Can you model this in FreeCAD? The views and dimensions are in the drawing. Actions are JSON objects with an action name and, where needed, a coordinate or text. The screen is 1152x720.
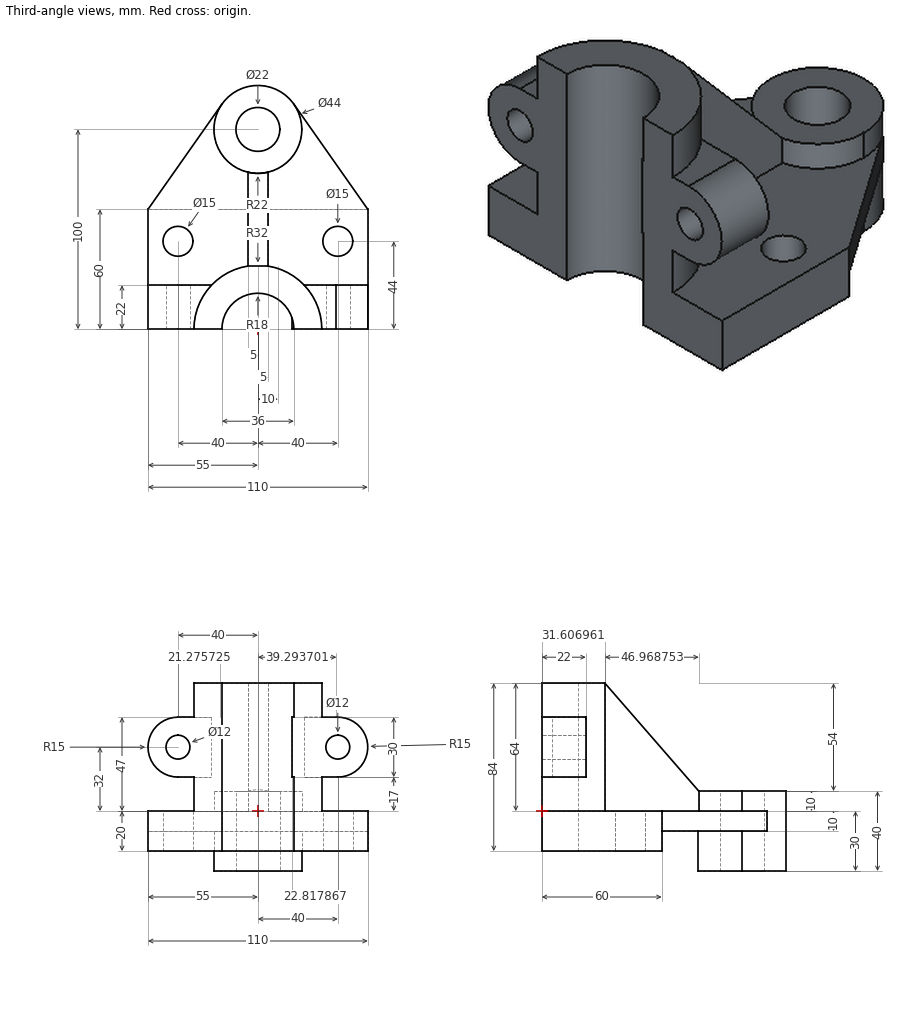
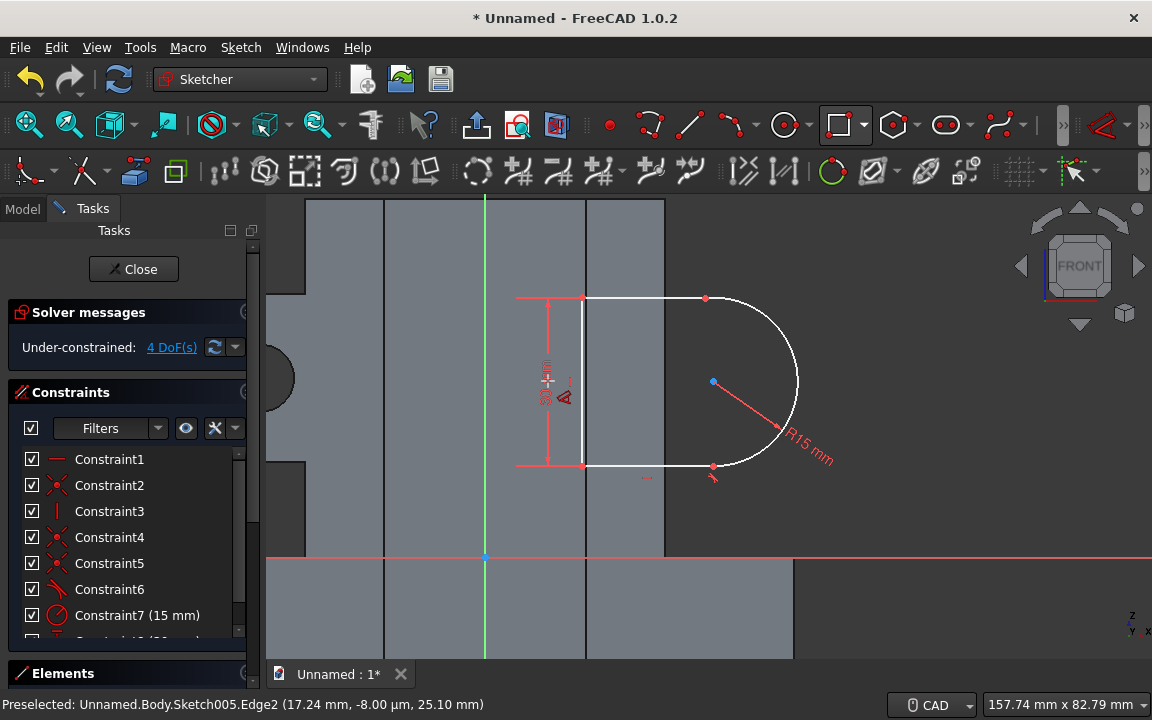
{"action": "left_click", "coordinate": [713, 466]}
{"action": "left_click", "coordinate": [599, 592]}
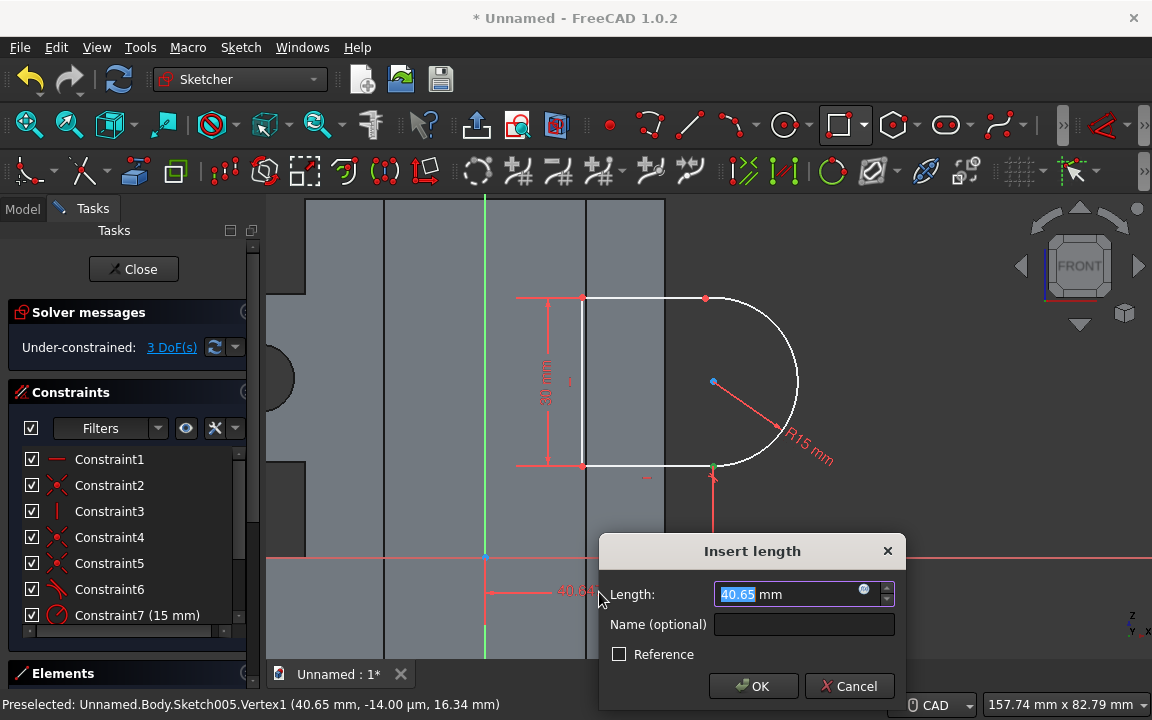
{"action": "type", "text": "40"}
{"action": "key", "text": "Return"}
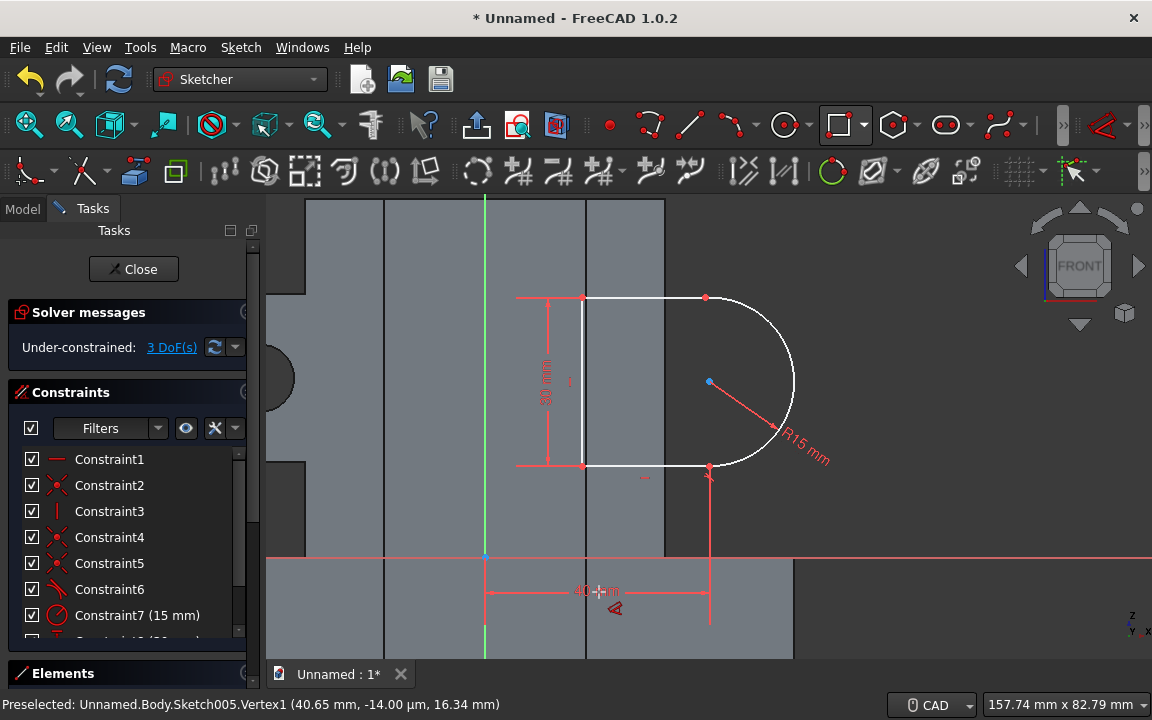
{"action": "left_click", "coordinate": [710, 466]}
{"action": "left_click", "coordinate": [451, 512]}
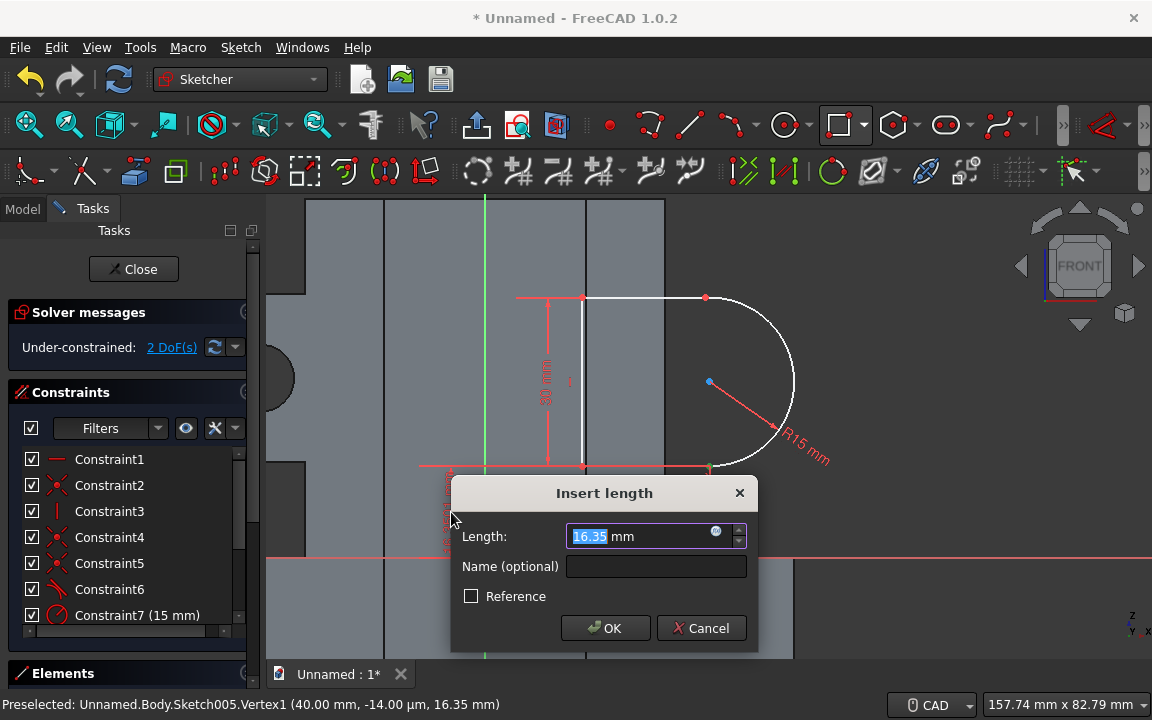
{"action": "type", "text": "17"}
{"action": "key", "text": "Return"}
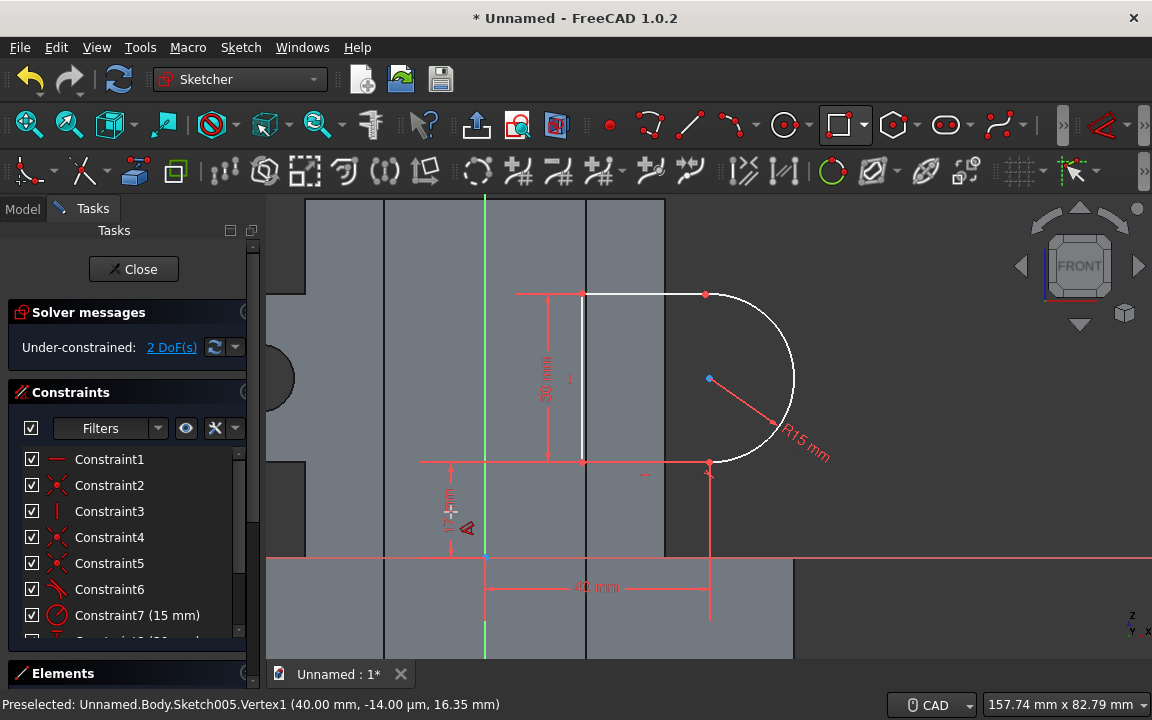
{"action": "left_click", "coordinate": [671, 462]}
{"action": "left_click", "coordinate": [646, 496]}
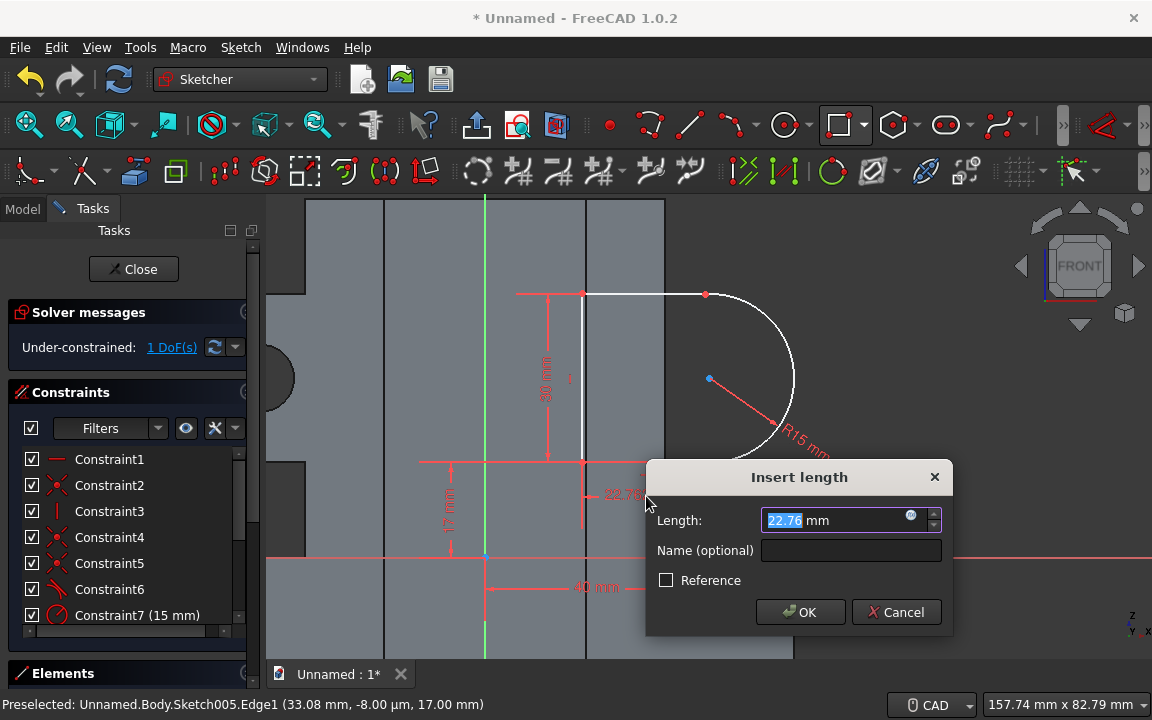
{"action": "type", "text": "22.817867"}
{"action": "key", "text": "Return"}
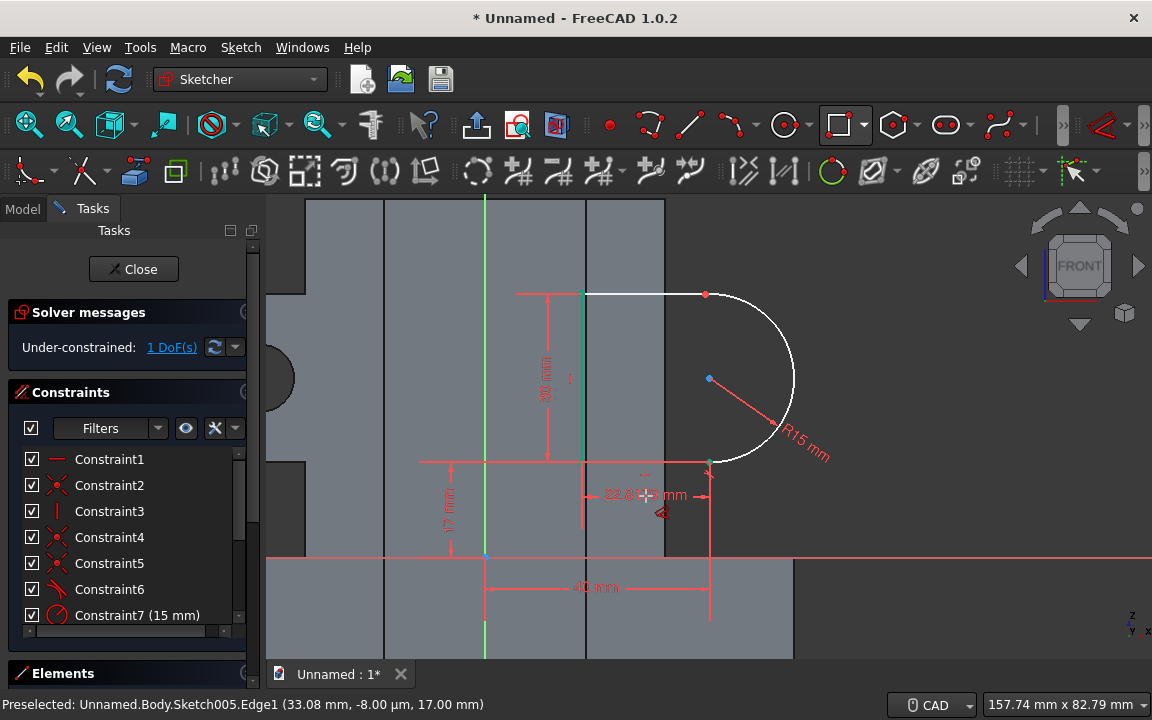
{"action": "left_click", "coordinate": [706, 294]}
{"action": "left_click", "coordinate": [518, 592]}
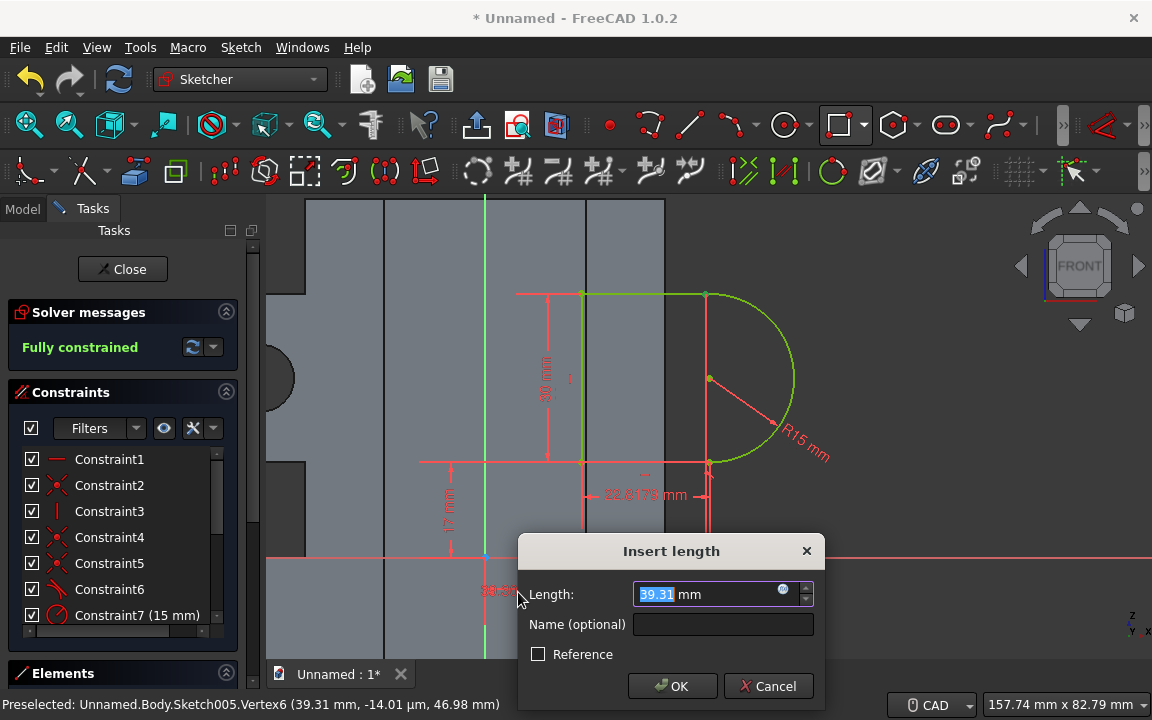
{"action": "type", "text": "39.293701"}
{"action": "key", "text": "Return"}
{"action": "key", "text": "Escape"}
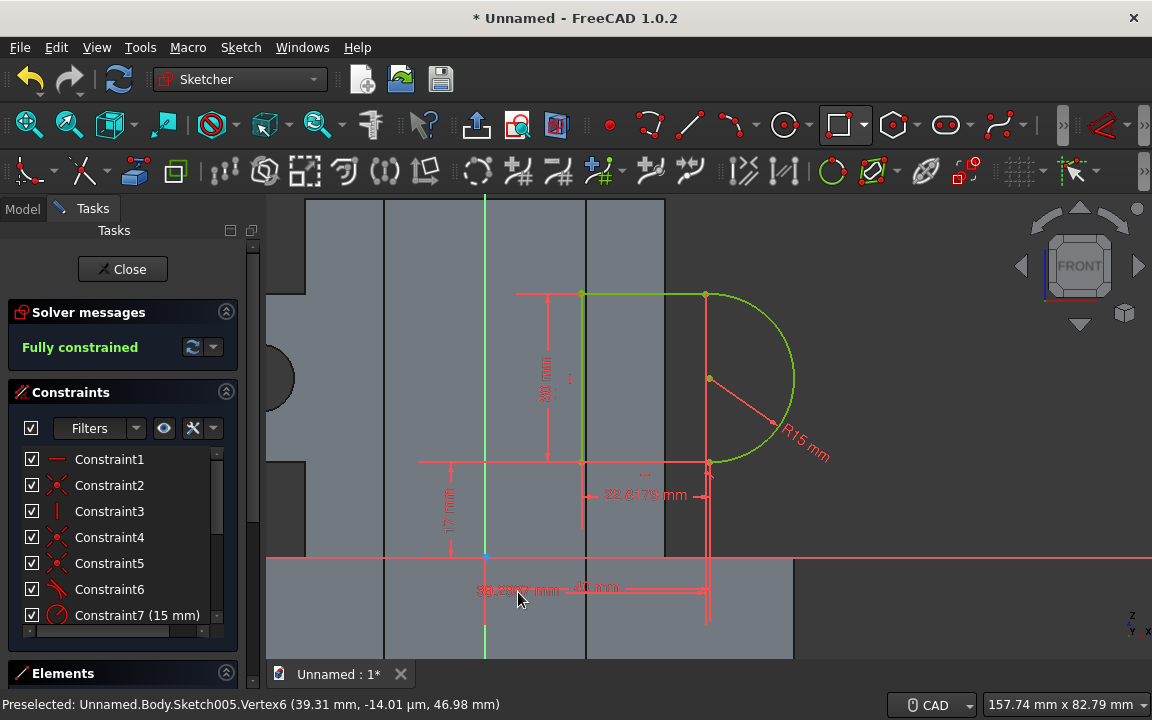
{"action": "left_click", "coordinate": [123, 269]}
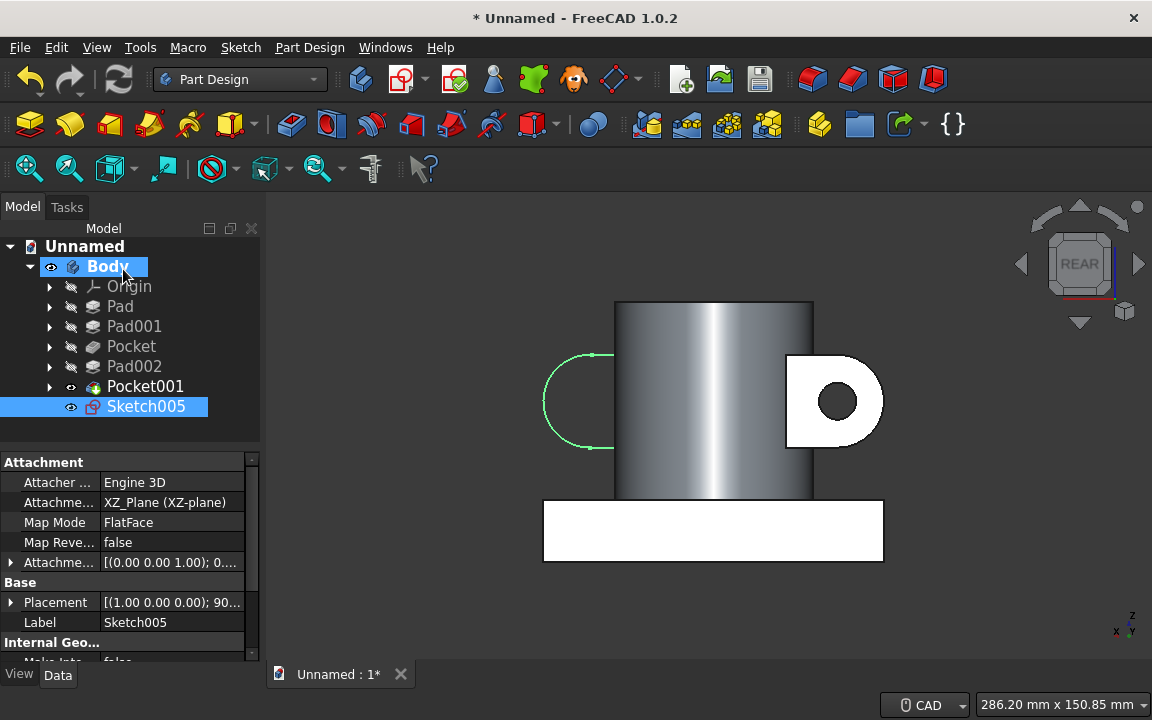
{"action": "left_click", "coordinate": [30, 124]}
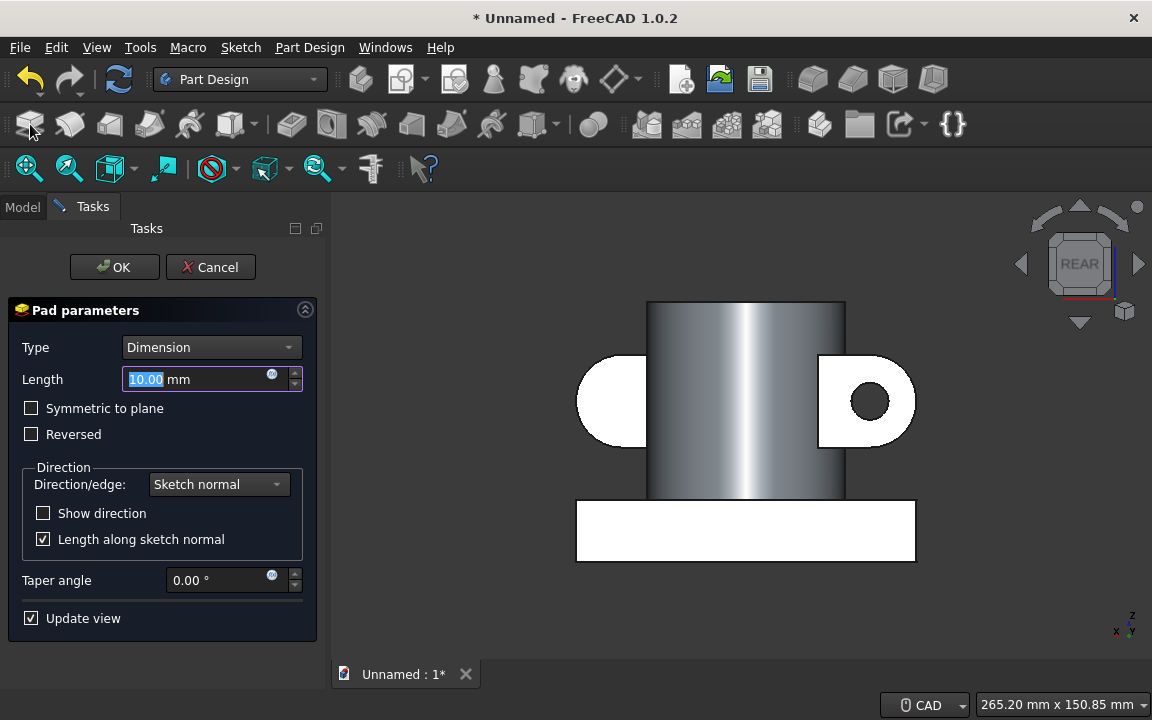
{"action": "type", "text": "22"}
{"action": "key", "text": "Tab"}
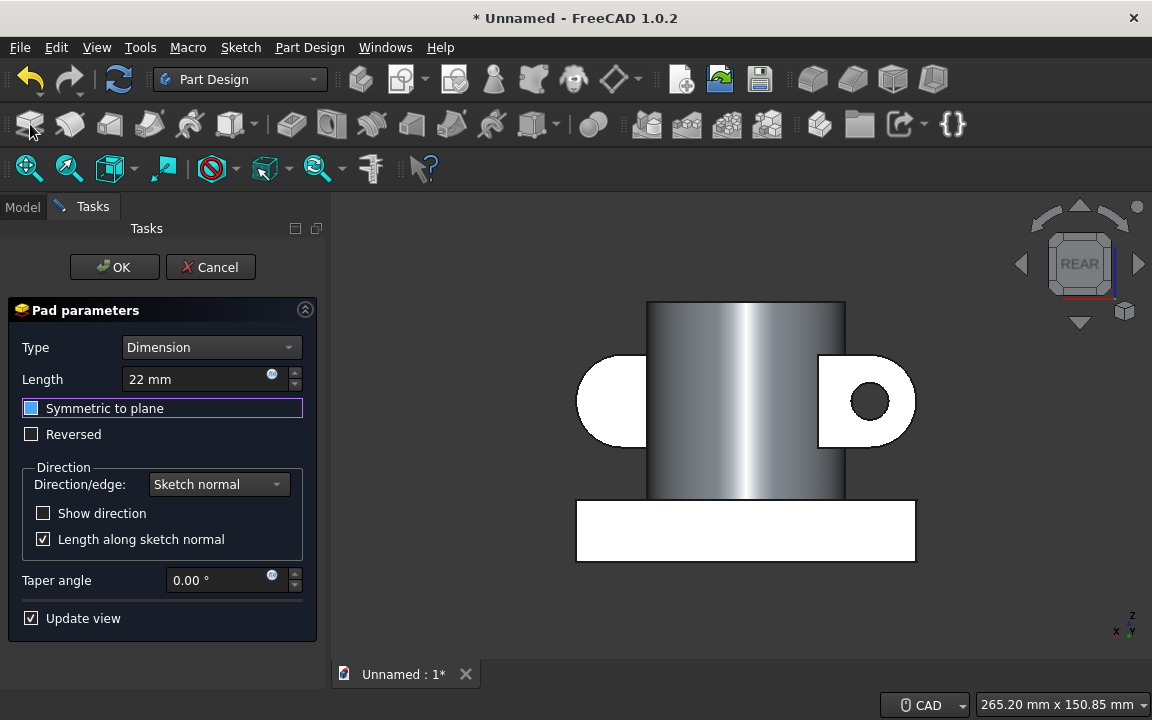
{"action": "left_click", "coordinate": [30, 434]}